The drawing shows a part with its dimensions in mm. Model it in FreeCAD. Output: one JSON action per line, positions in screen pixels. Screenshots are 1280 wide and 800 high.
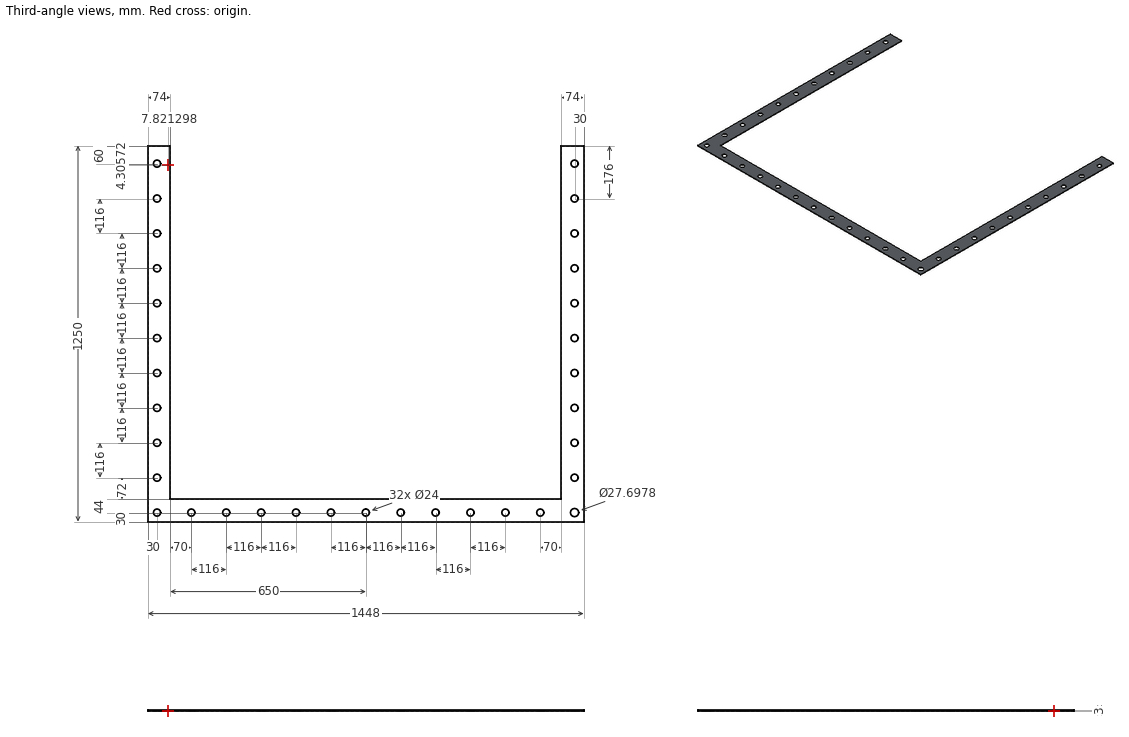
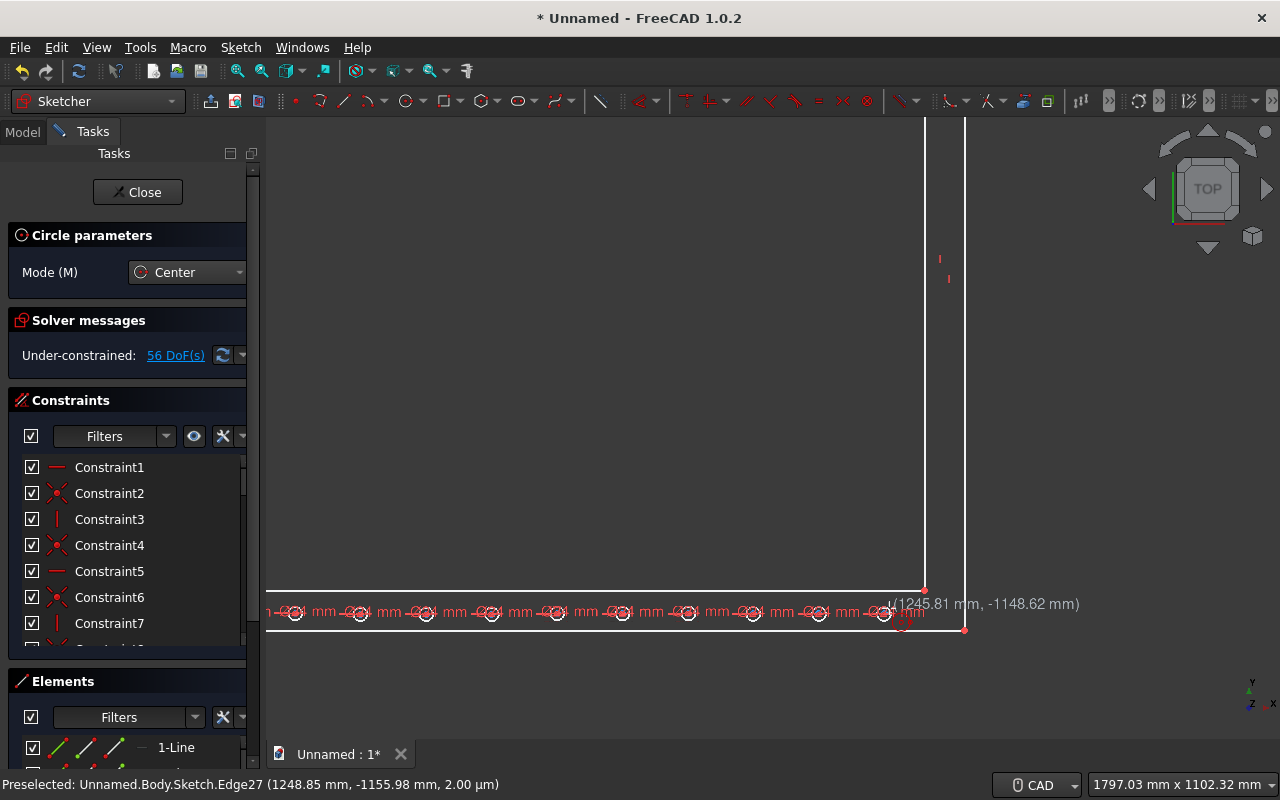
{"action": "scroll", "coordinate": [949, 613], "scroll_direction": "up", "scroll_amount": 6}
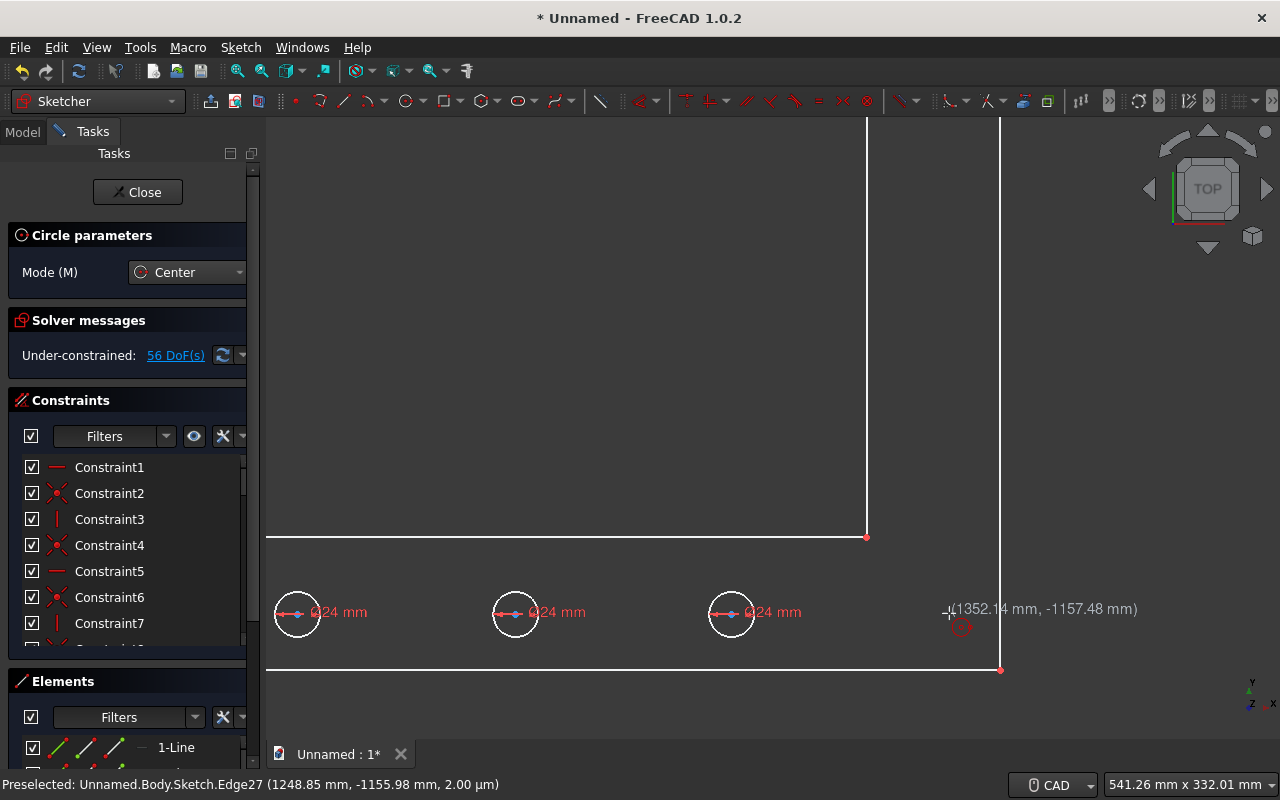
{"action": "scroll", "coordinate": [914, 612], "scroll_direction": "down", "scroll_amount": 9}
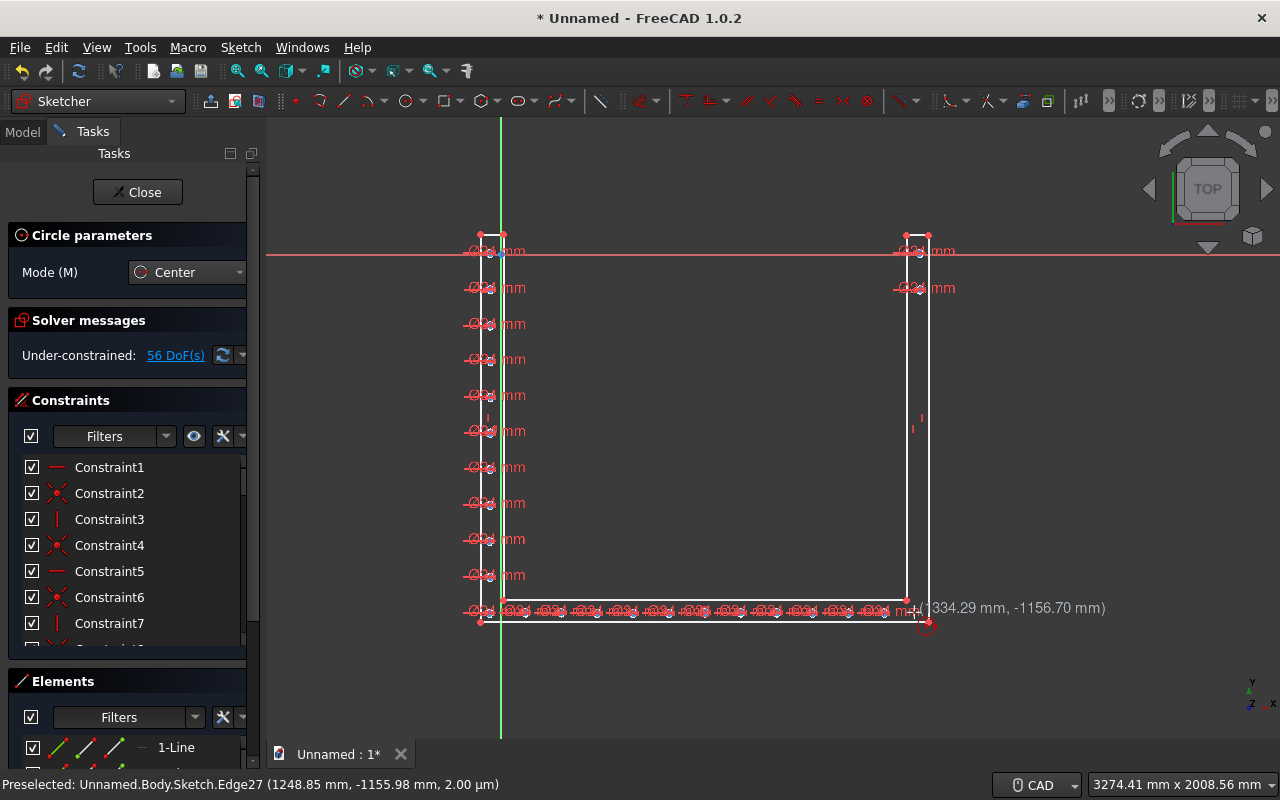
{"action": "scroll", "coordinate": [920, 613], "scroll_direction": "up", "scroll_amount": 3}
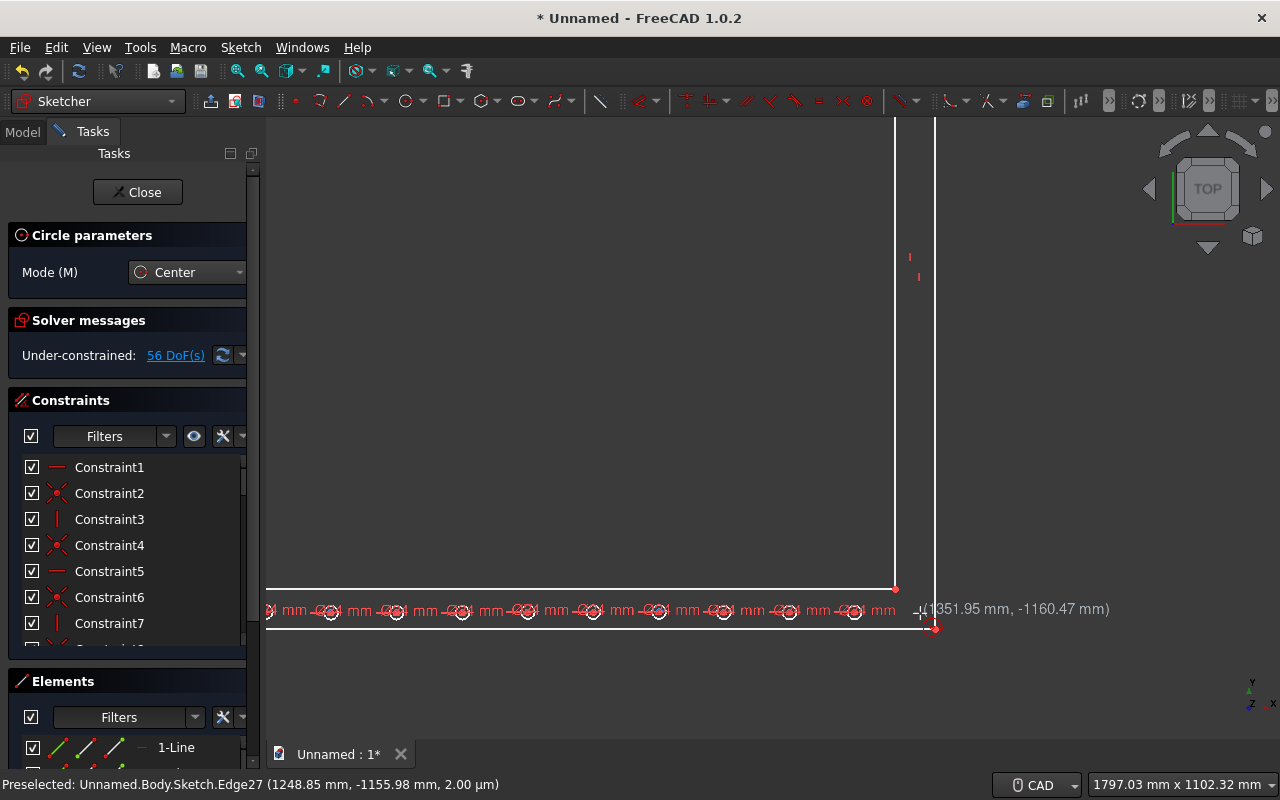
{"action": "left_click", "coordinate": [919, 611]}
{"action": "mouse_move", "coordinate": [914, 606]}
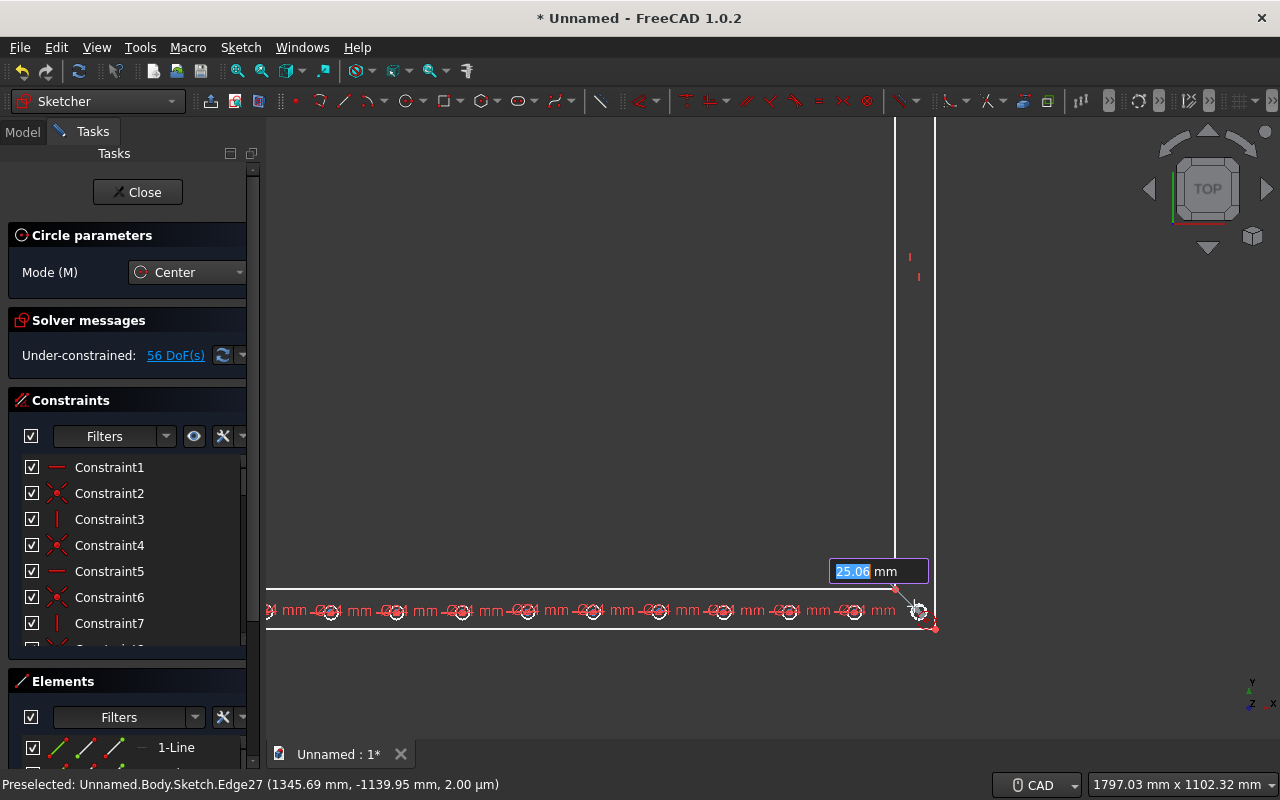
{"action": "type", "text": "27.6978"}
{"action": "key", "text": "Return"}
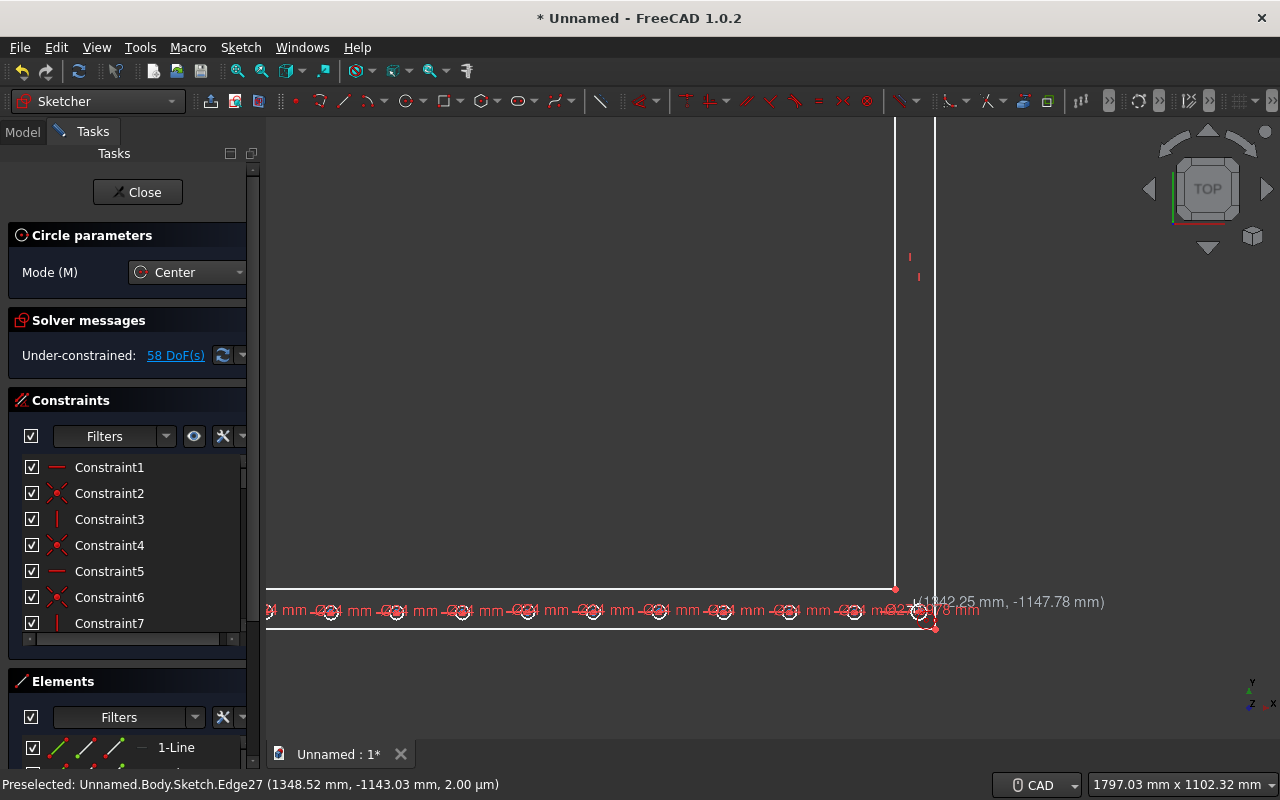
{"action": "scroll", "coordinate": [919, 546], "scroll_direction": "up", "scroll_amount": 7}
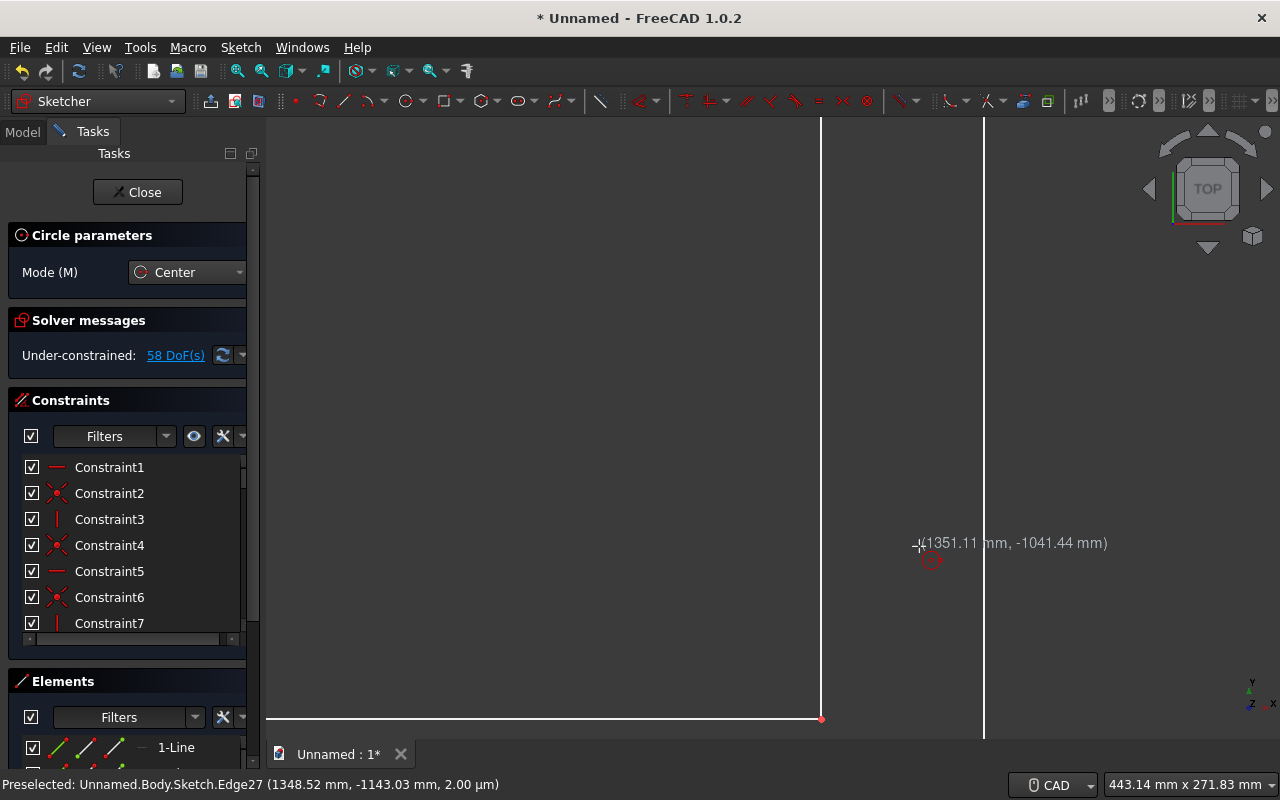
{"action": "scroll", "coordinate": [920, 581], "scroll_direction": "down", "scroll_amount": 10}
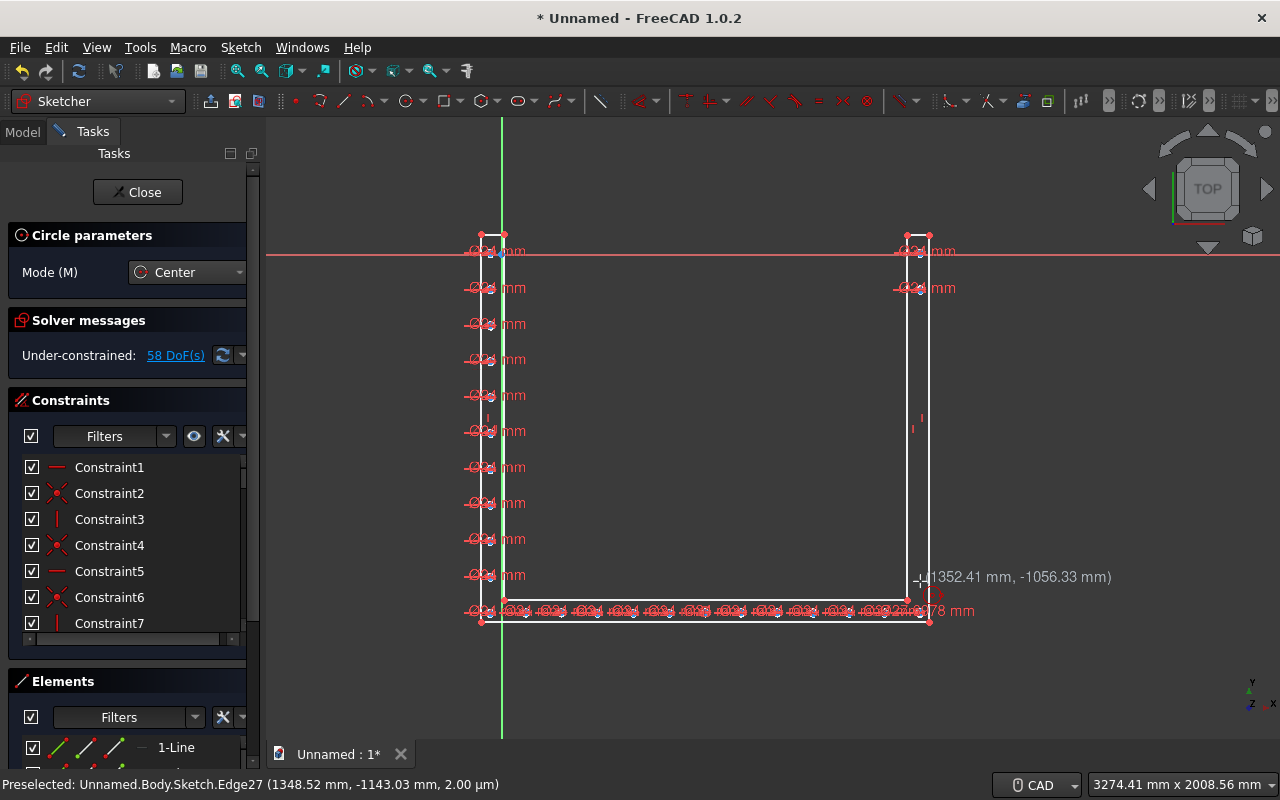
{"action": "scroll", "coordinate": [920, 577], "scroll_direction": "up", "scroll_amount": 3}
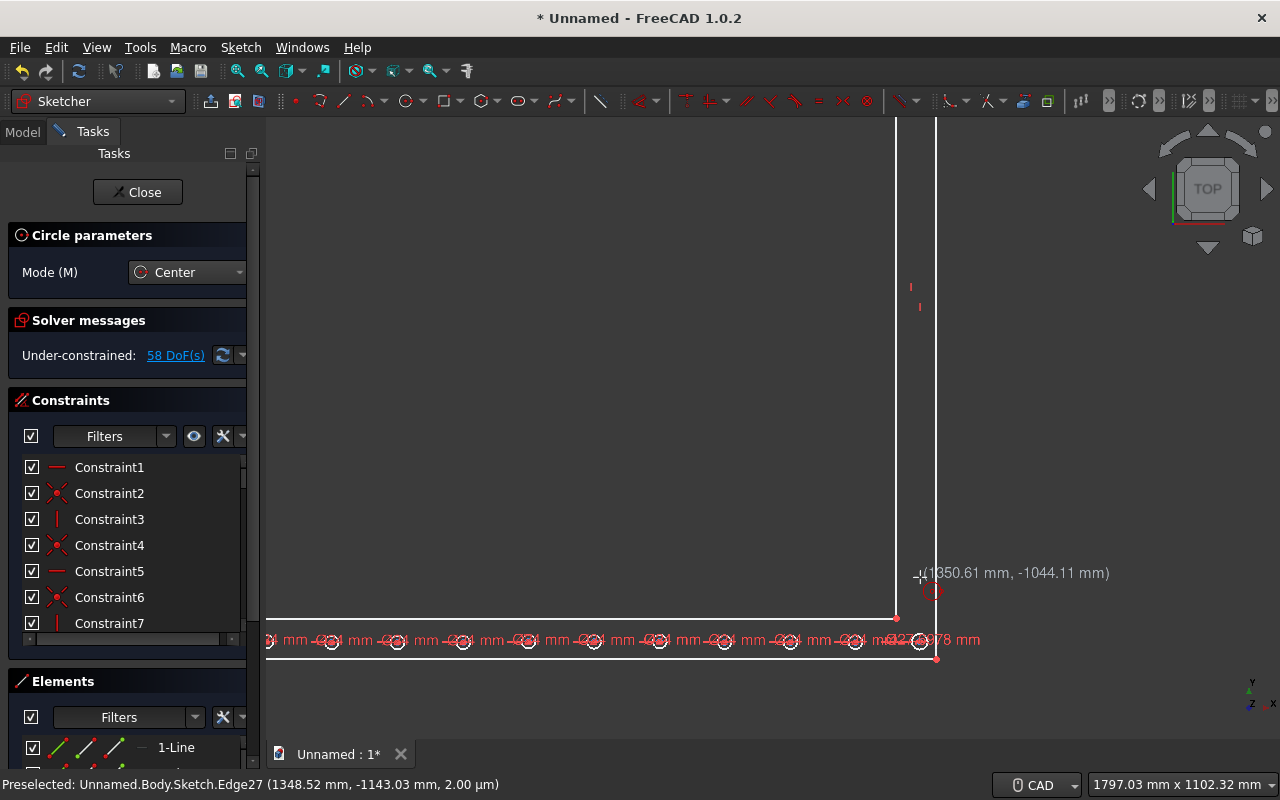
{"action": "left_click", "coordinate": [920, 576]}
{"action": "mouse_move", "coordinate": [915, 571]}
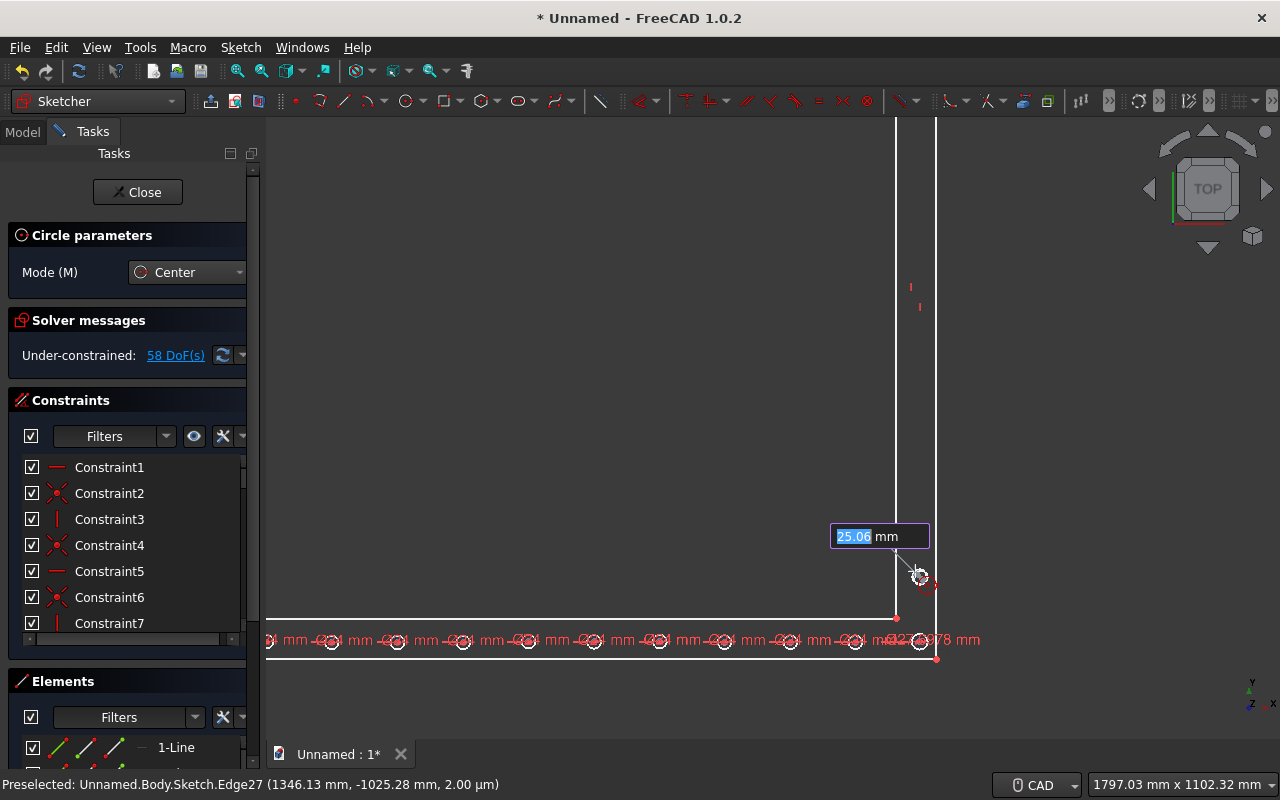
{"action": "type", "text": "24"}
{"action": "key", "text": "Return"}